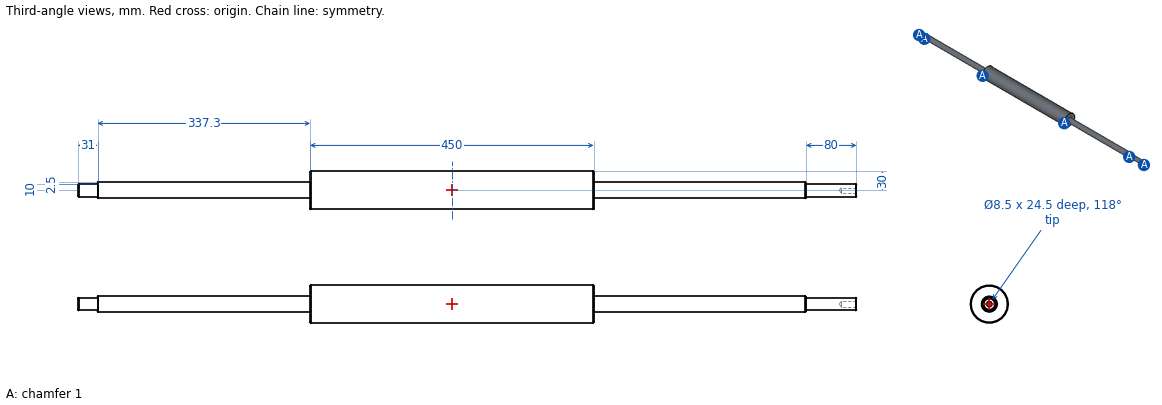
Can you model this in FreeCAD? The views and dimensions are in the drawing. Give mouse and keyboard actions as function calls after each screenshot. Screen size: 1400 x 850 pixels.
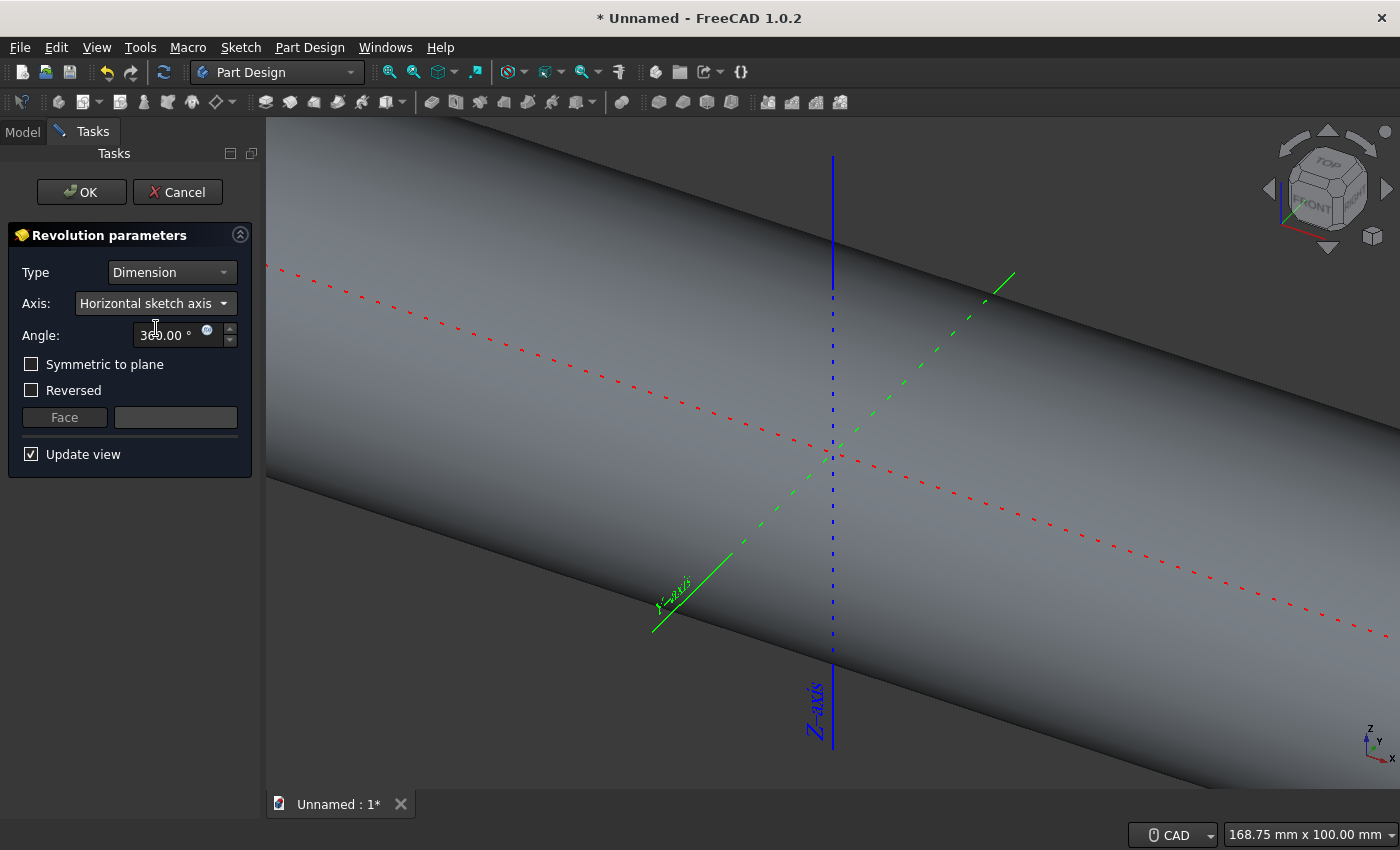
click(82, 192)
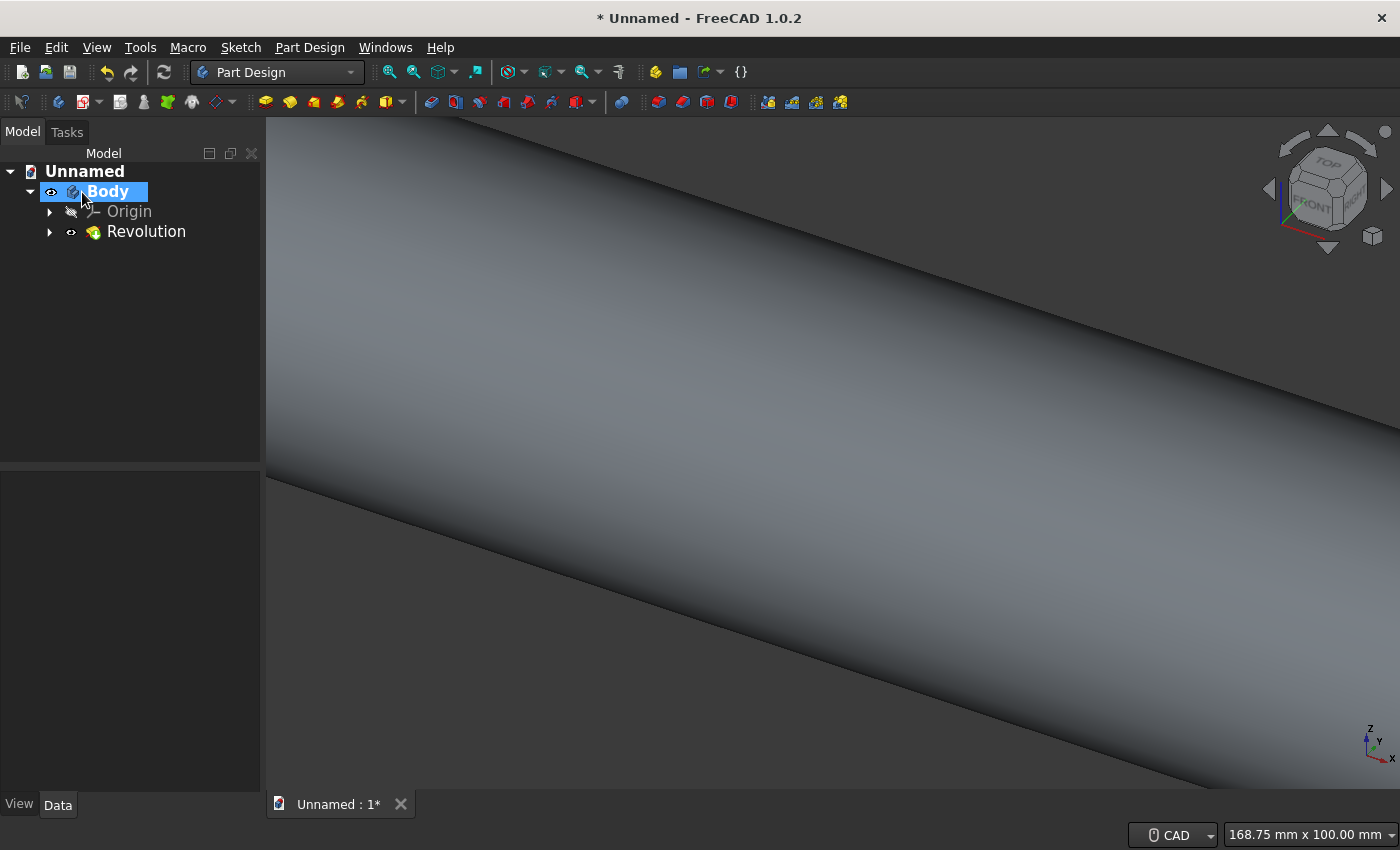
key(v)
key(f)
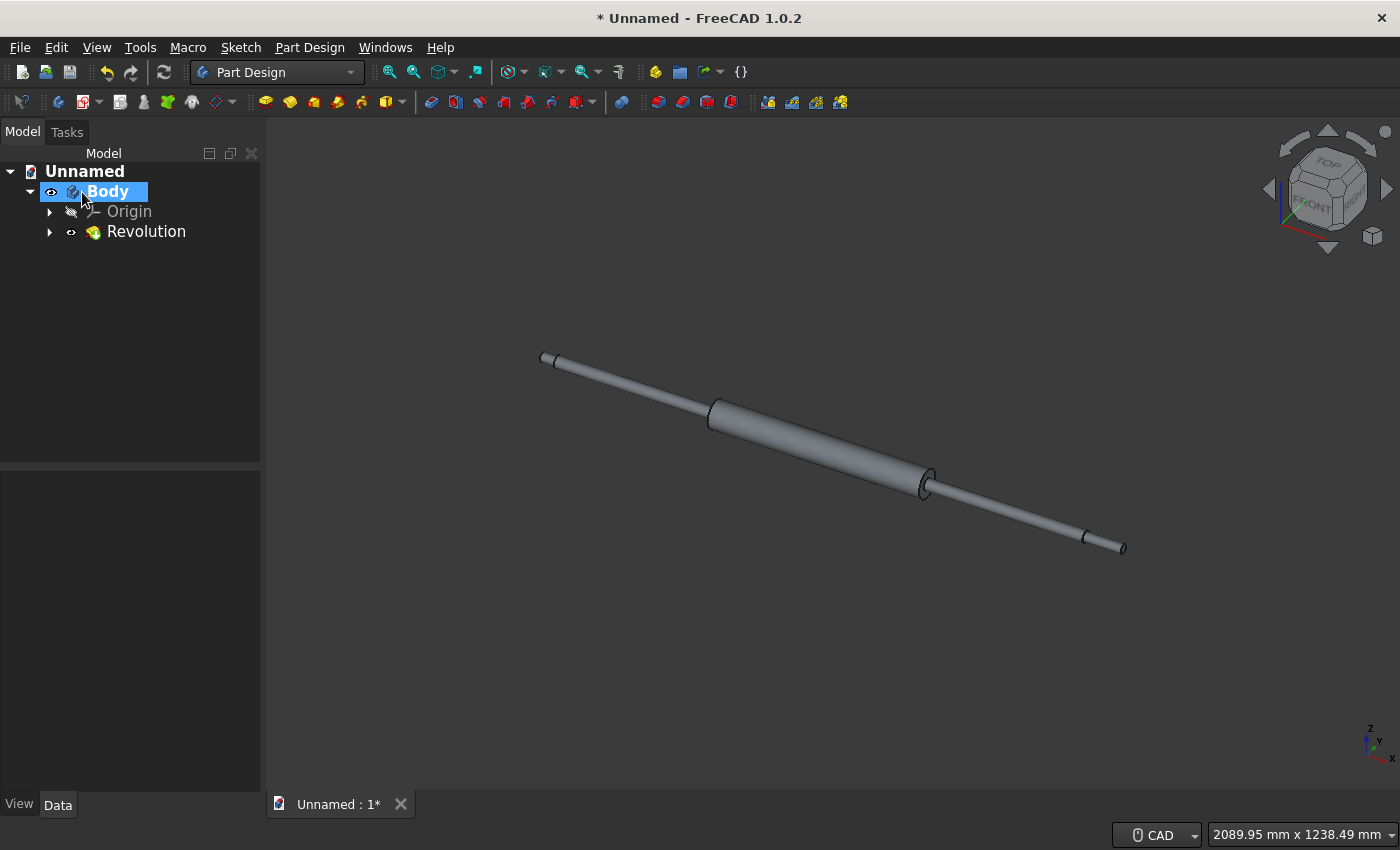
click(919, 491)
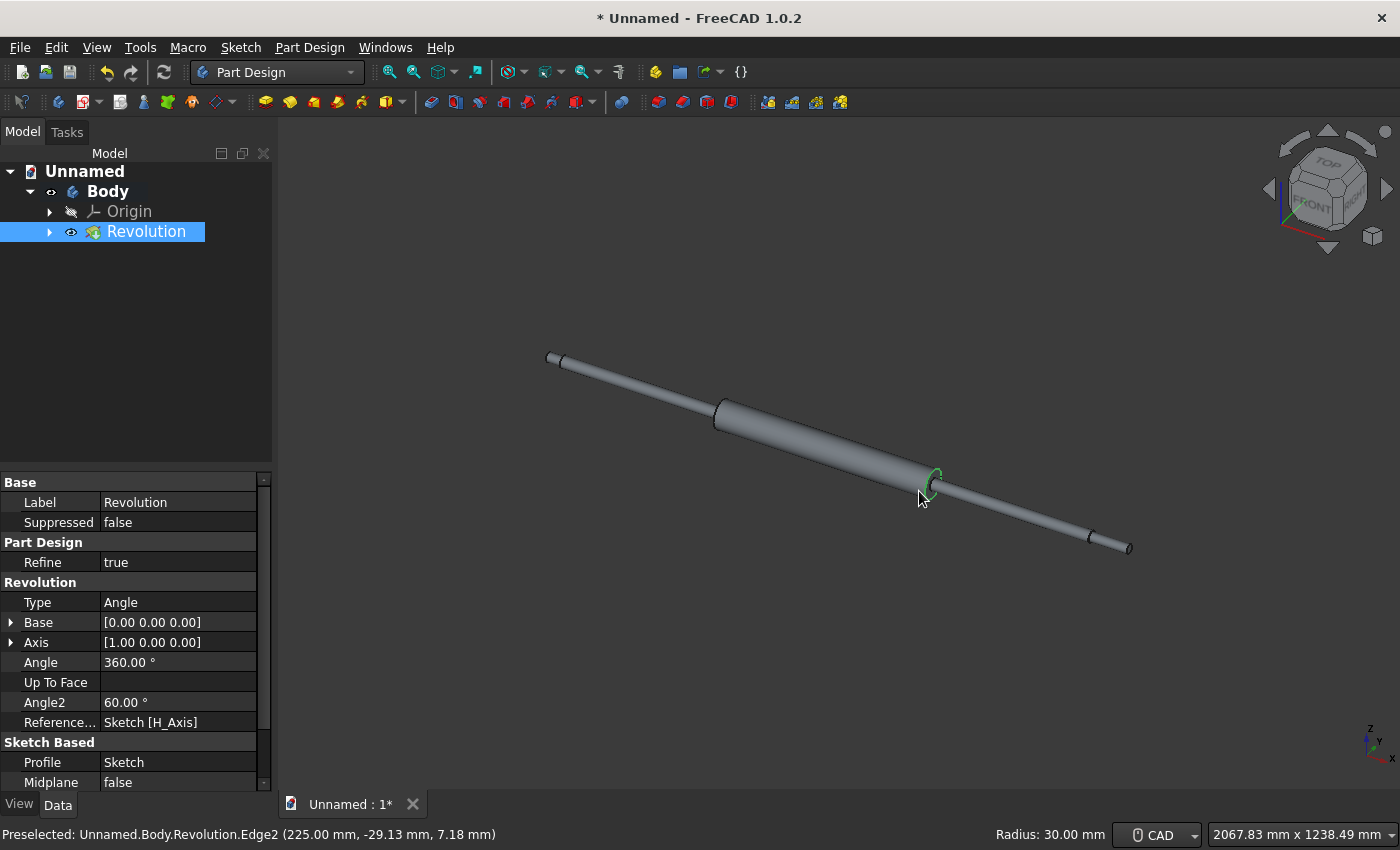
click(714, 421, ctrl)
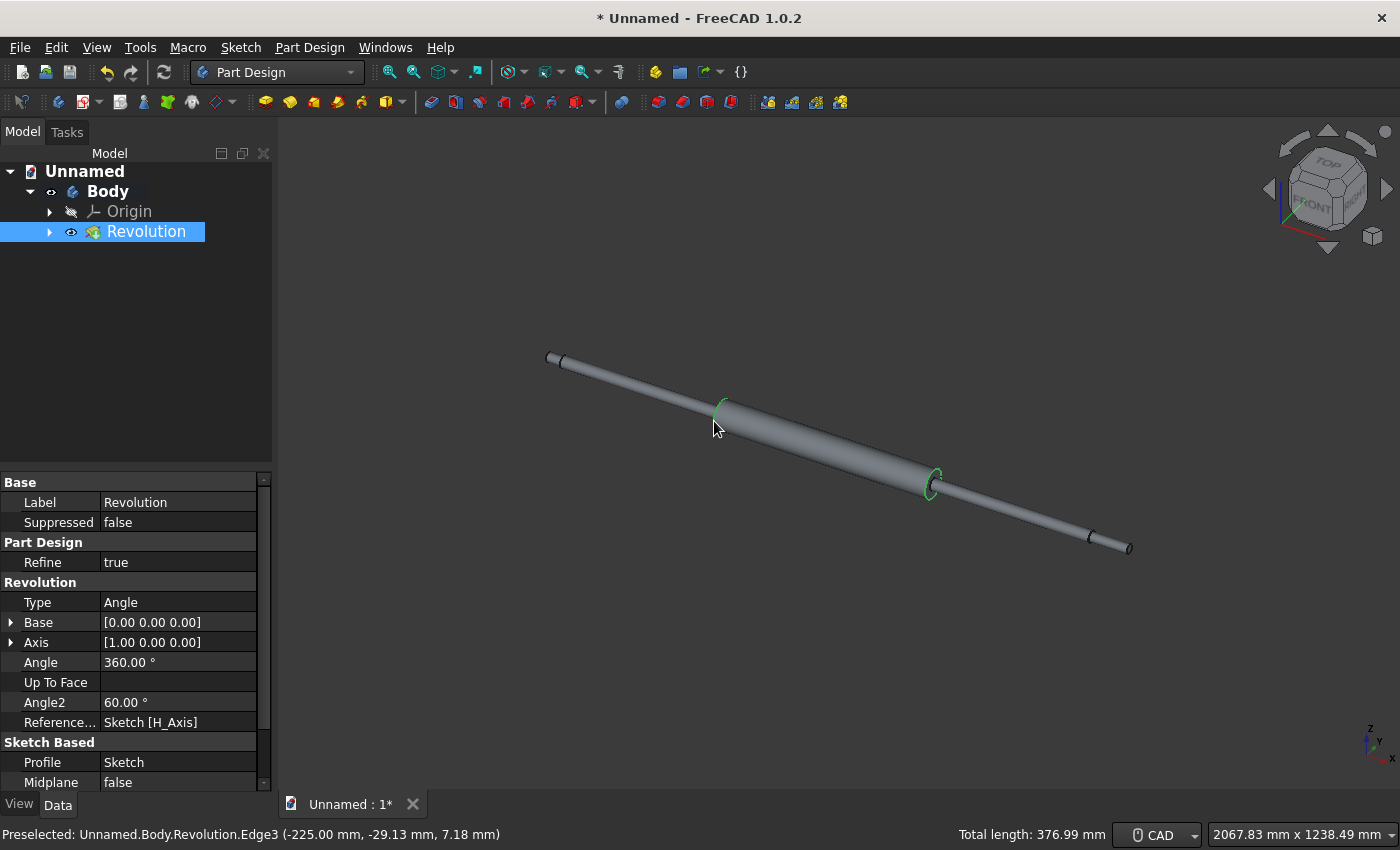
click(560, 364, ctrl)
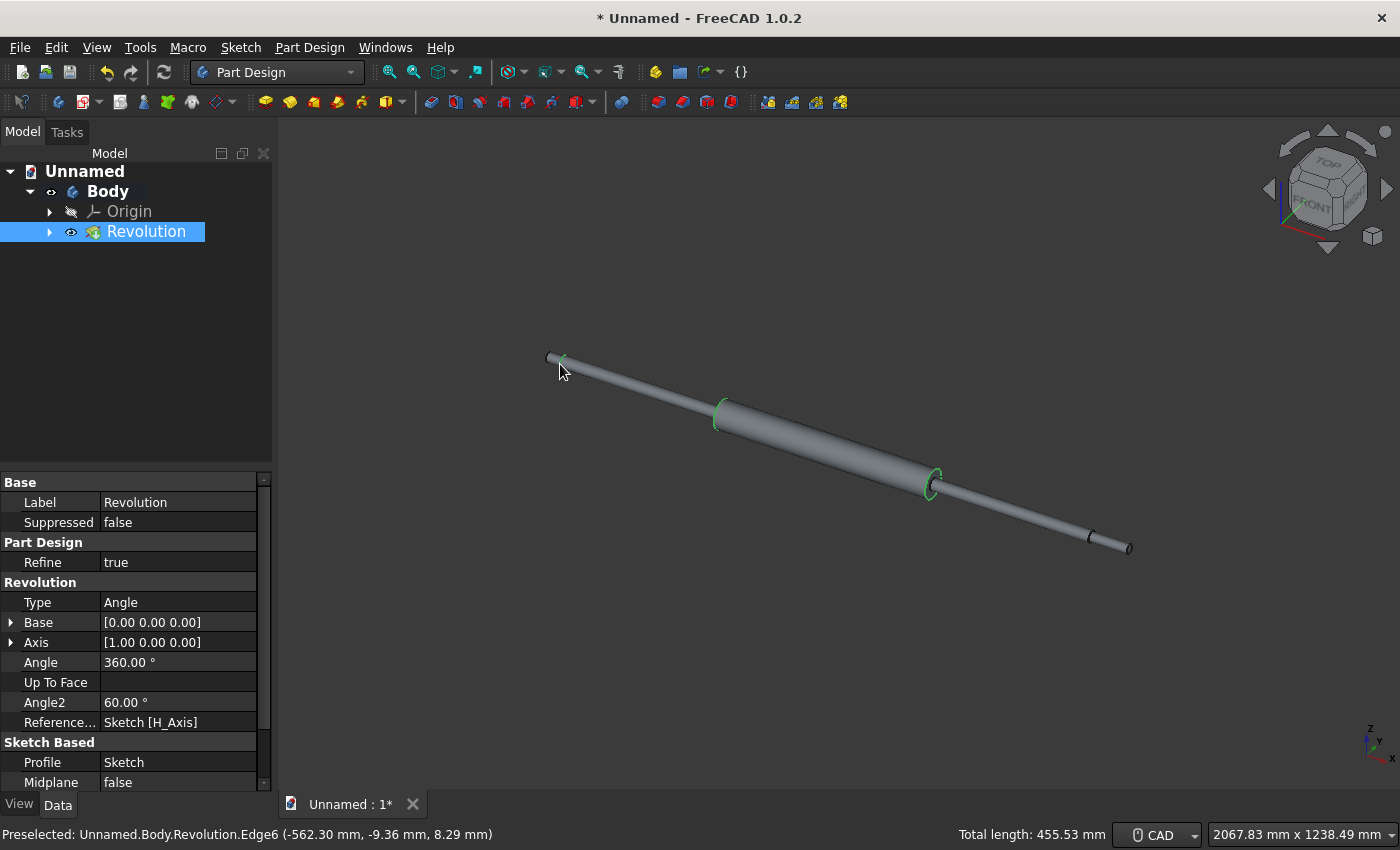
click(546, 359, ctrl)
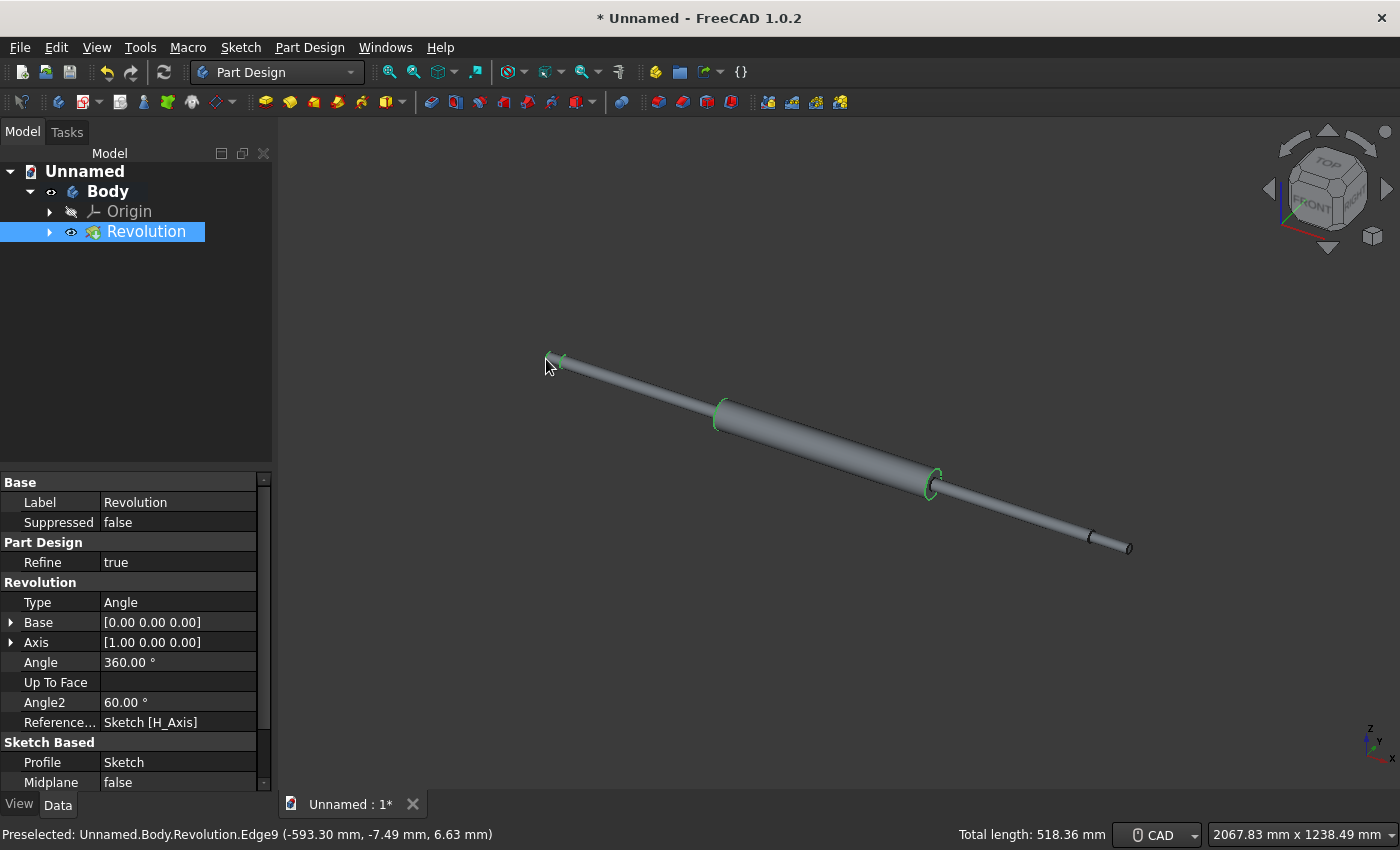
click(1127, 551, ctrl)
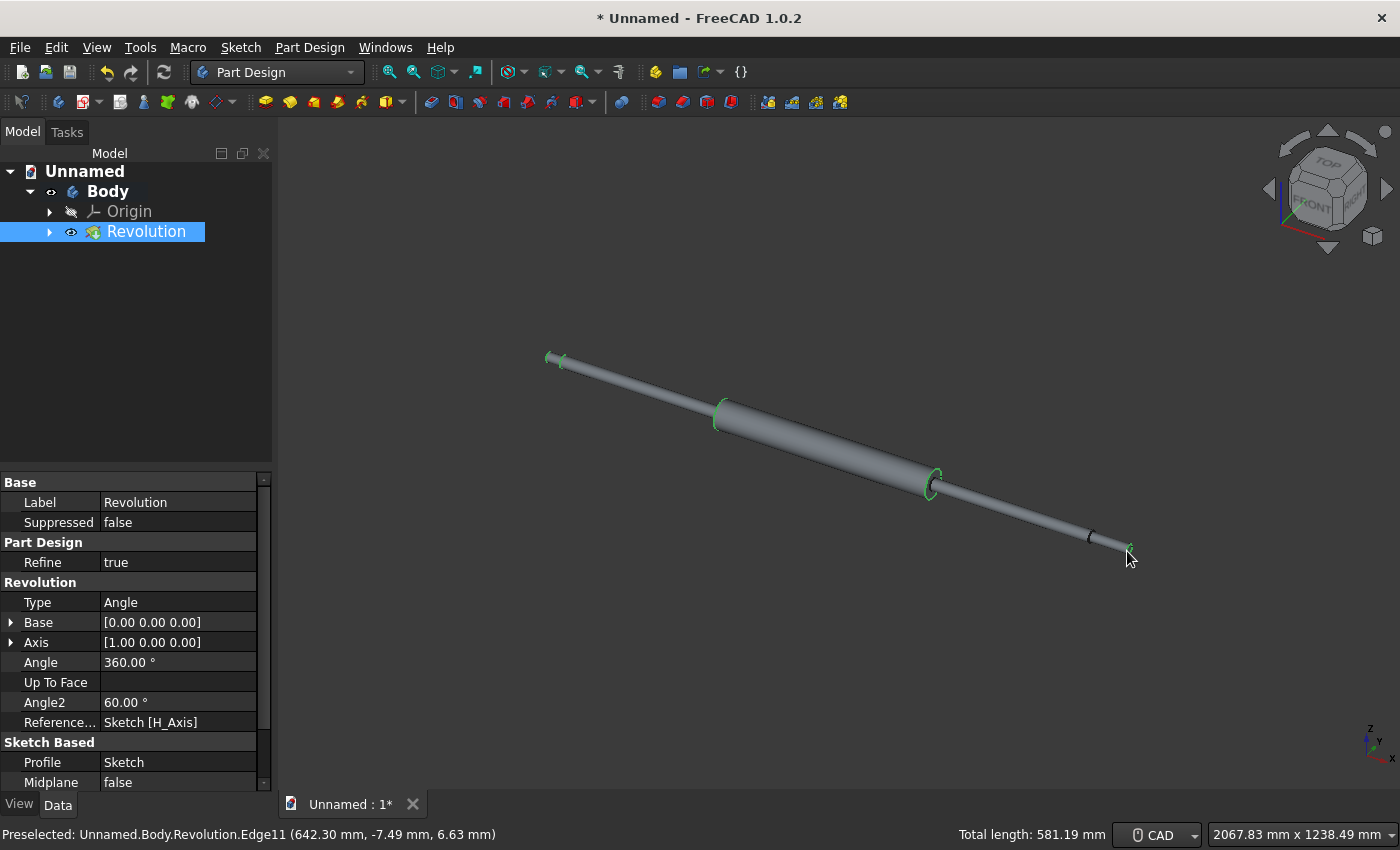
click(1088, 539, ctrl)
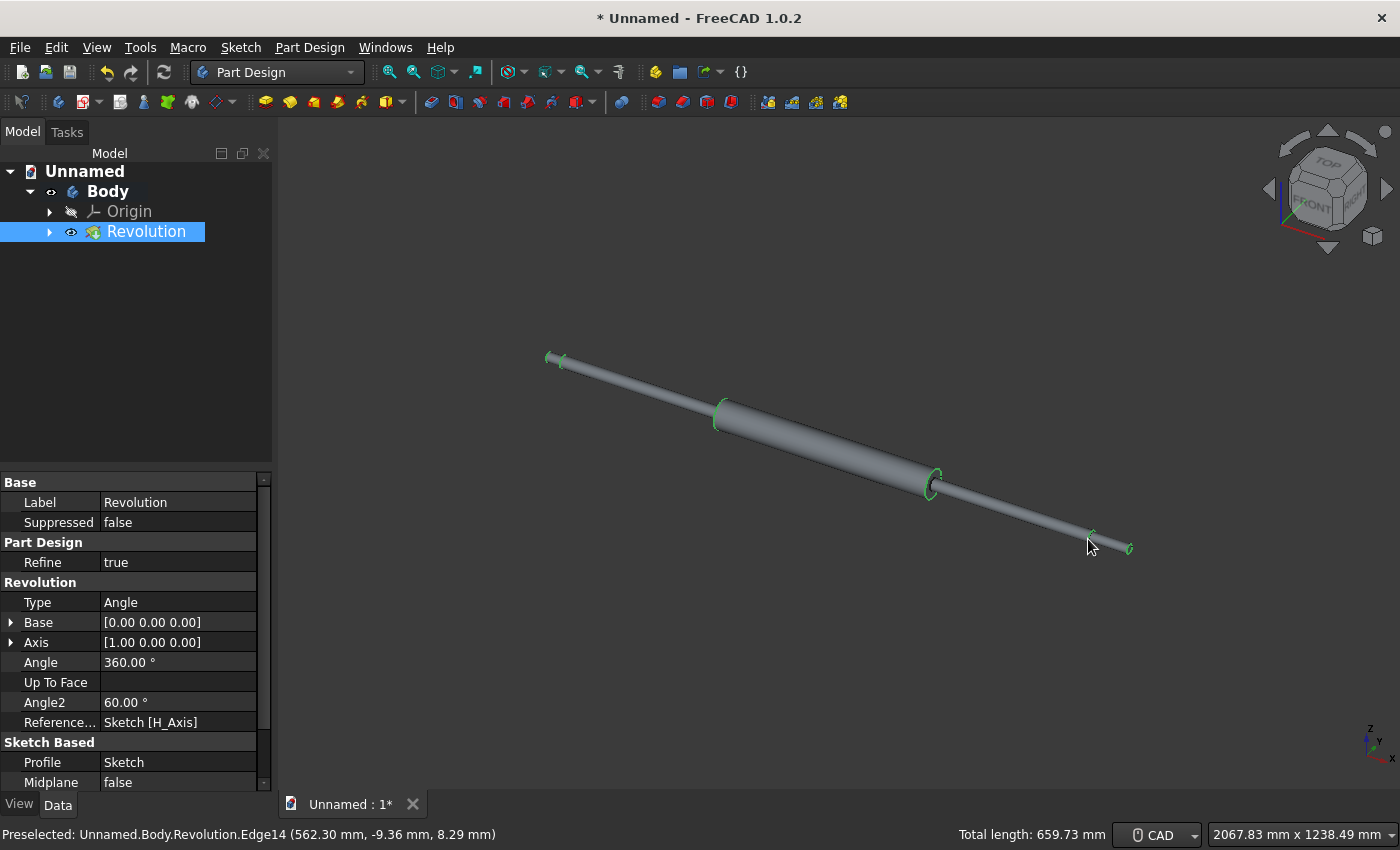
click(684, 102)